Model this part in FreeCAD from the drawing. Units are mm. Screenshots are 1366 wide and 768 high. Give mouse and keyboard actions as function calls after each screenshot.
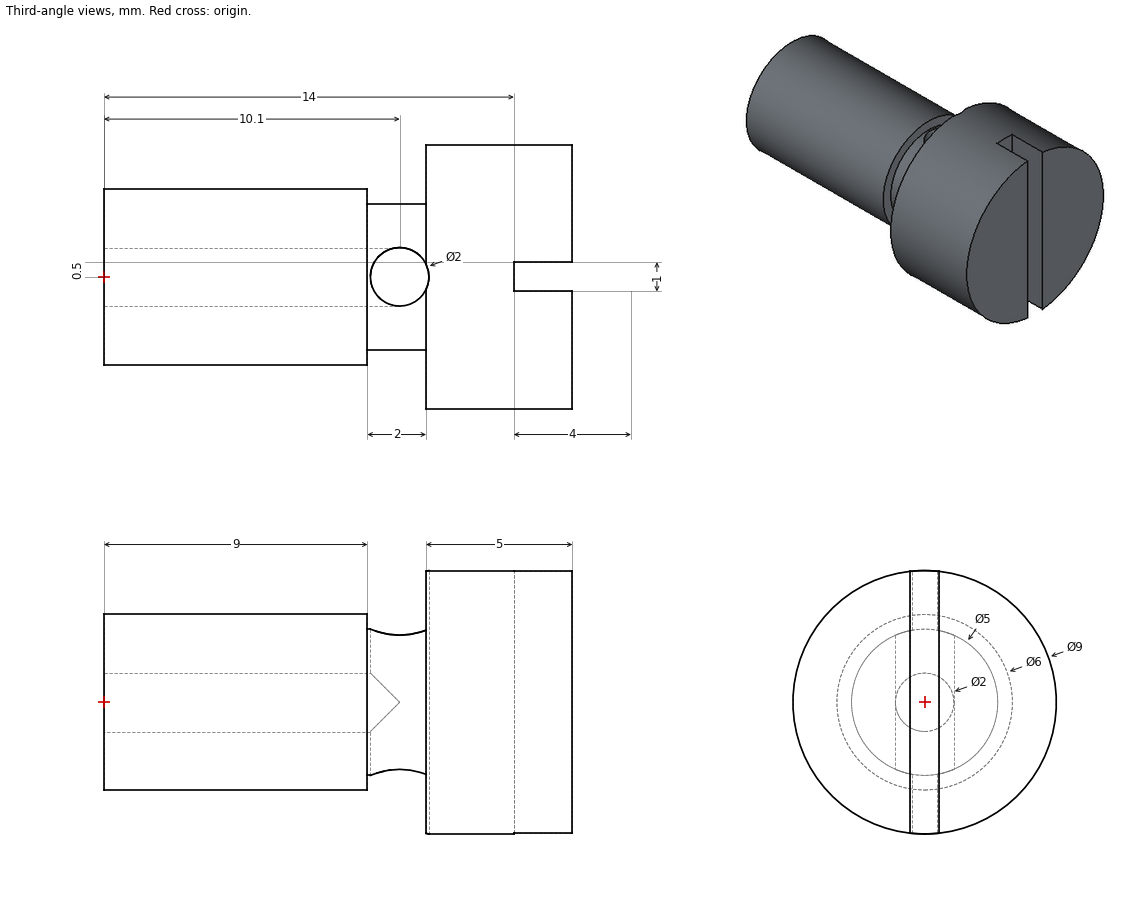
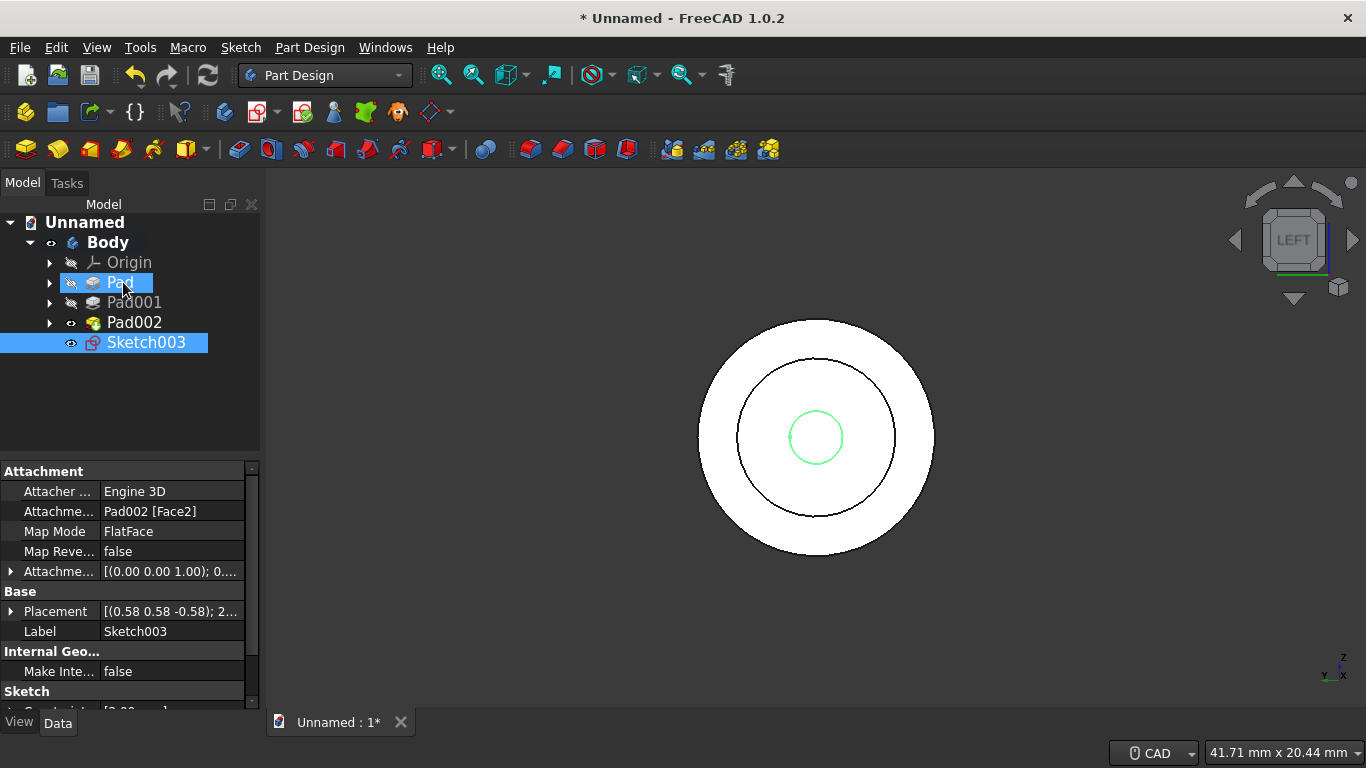
click(240, 150)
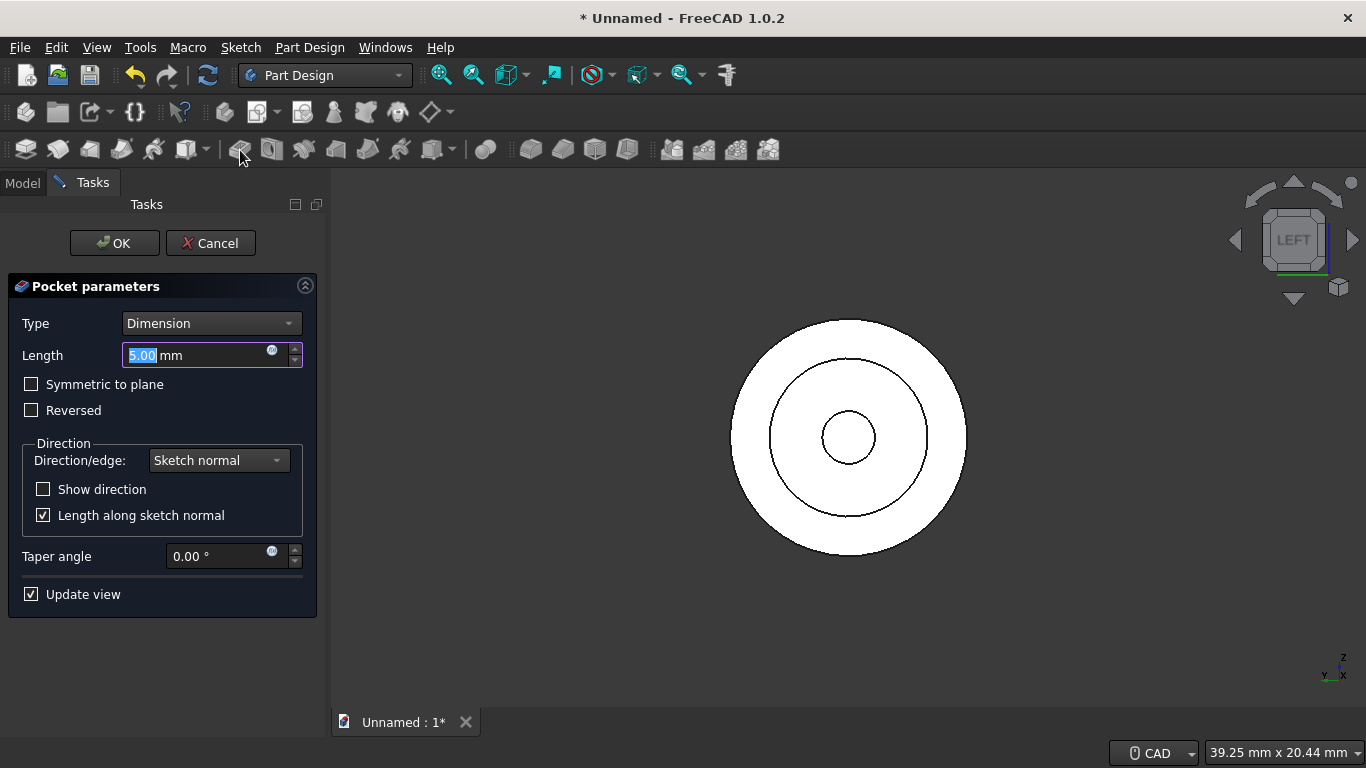
click(212, 324)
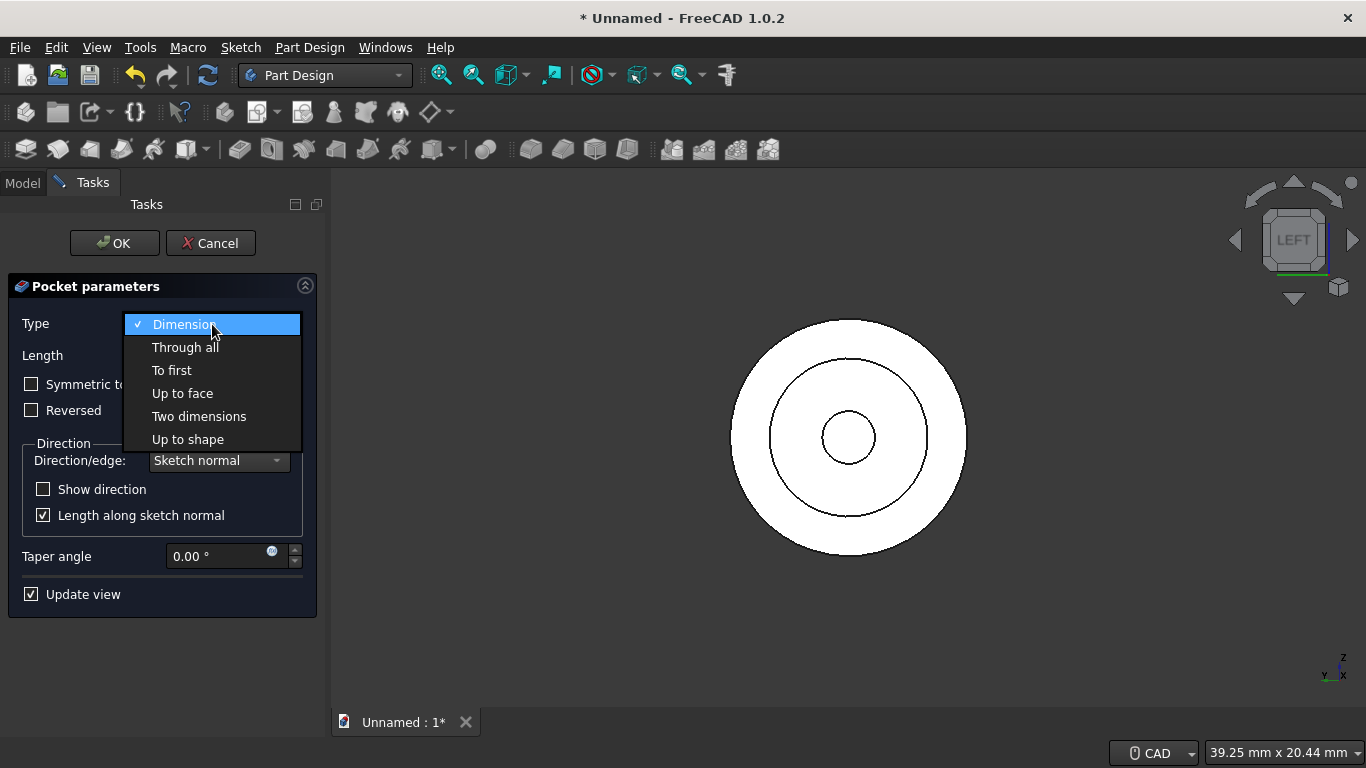
click(212, 416)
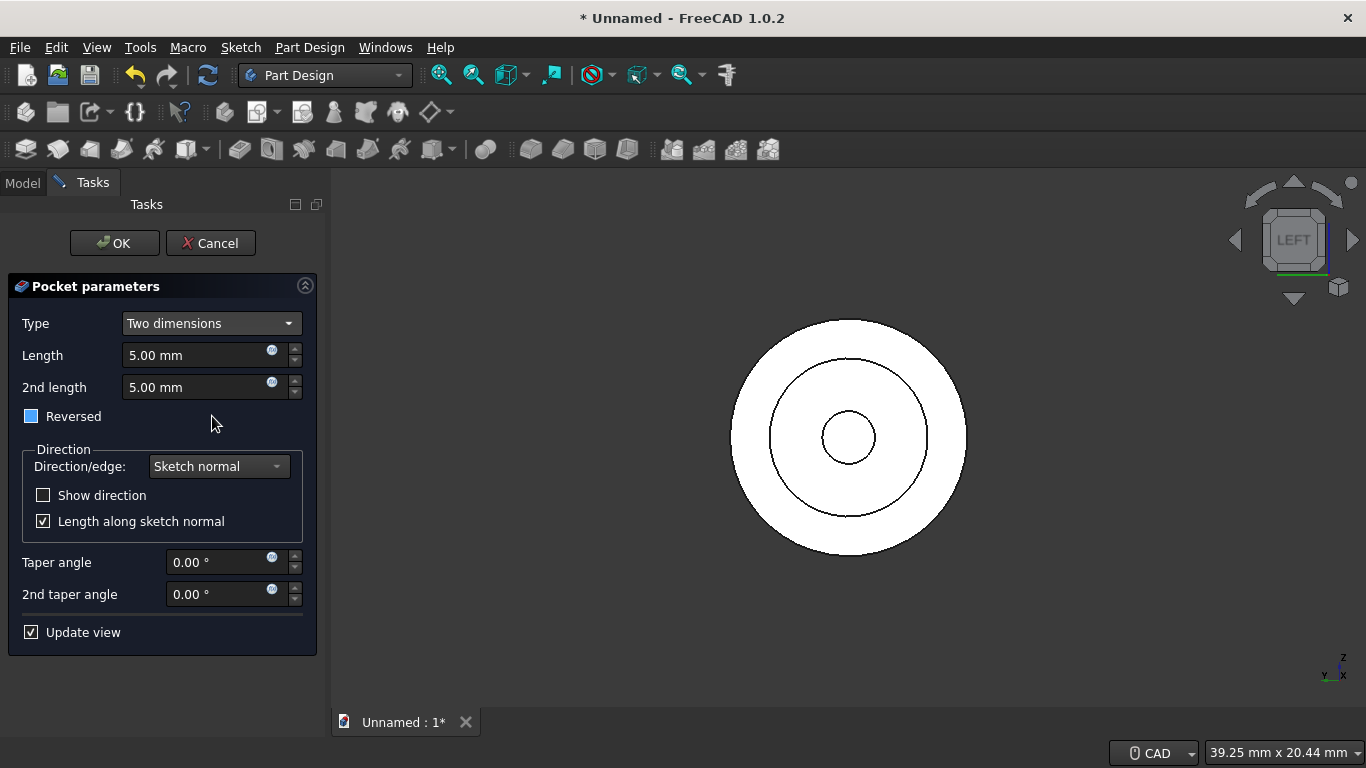
triple_click(204, 355)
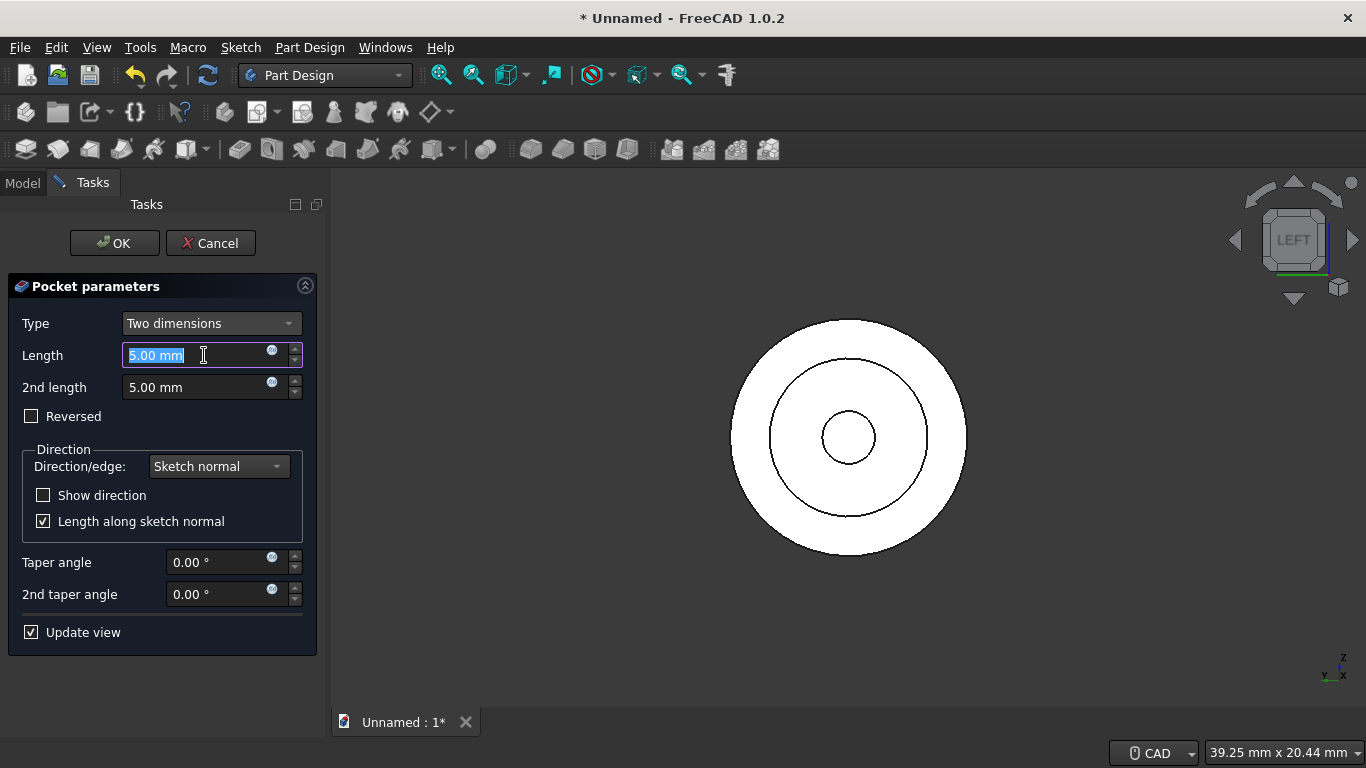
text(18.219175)
key(Tab)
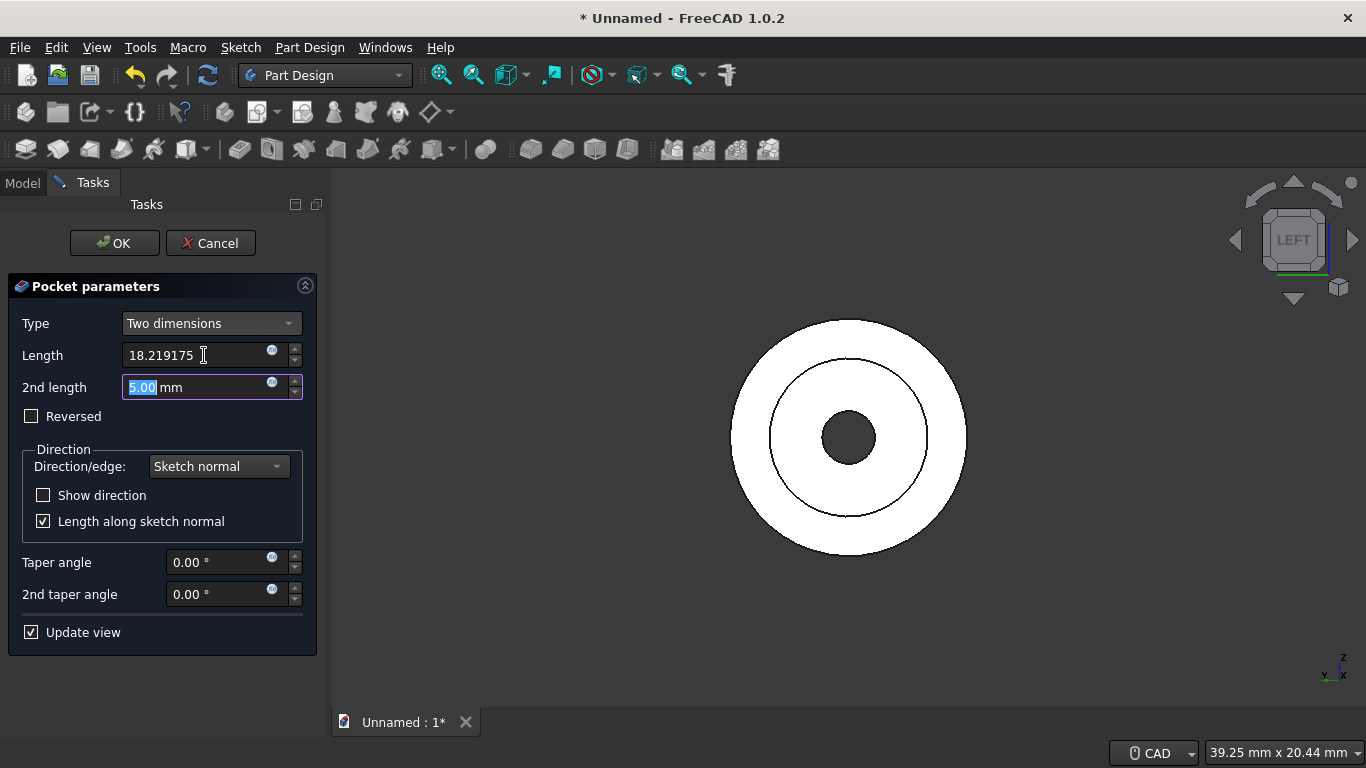
text(10.1)
key(Tab)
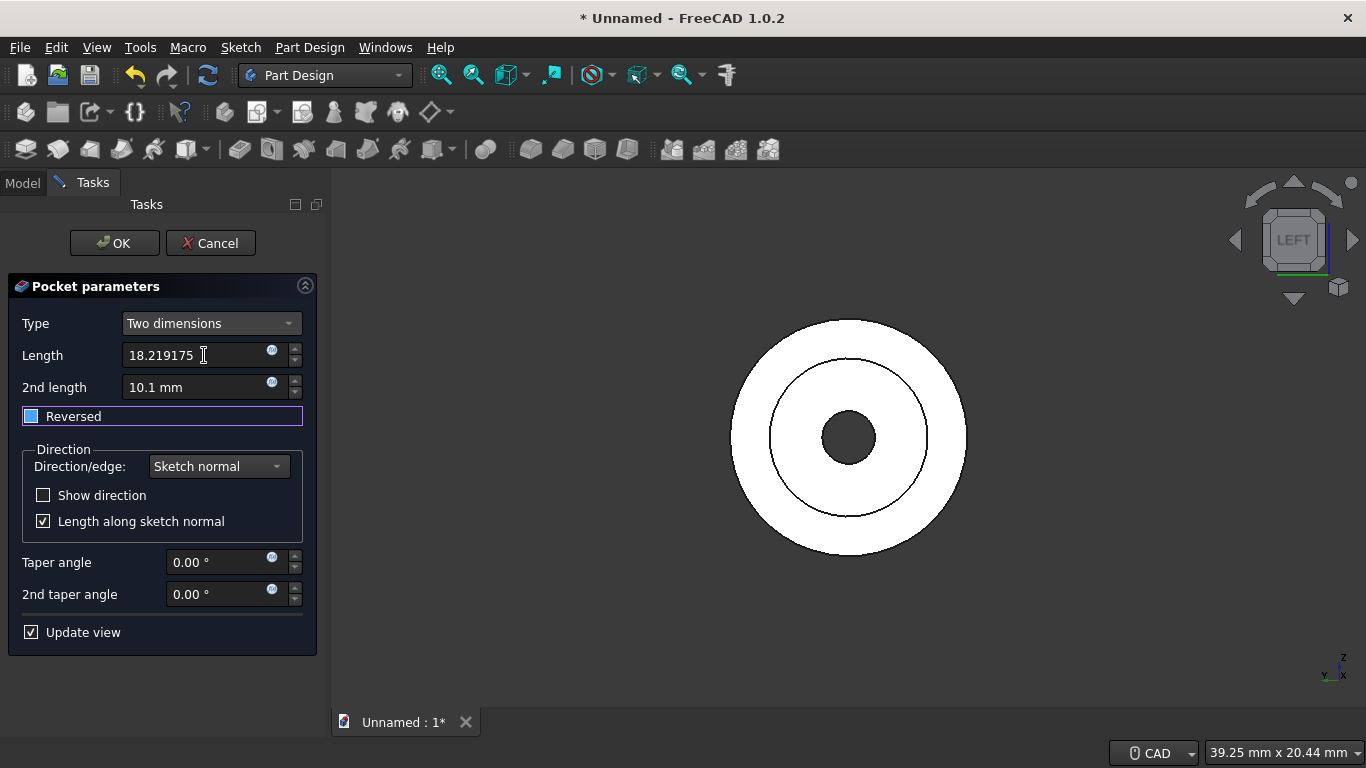
click(30, 416)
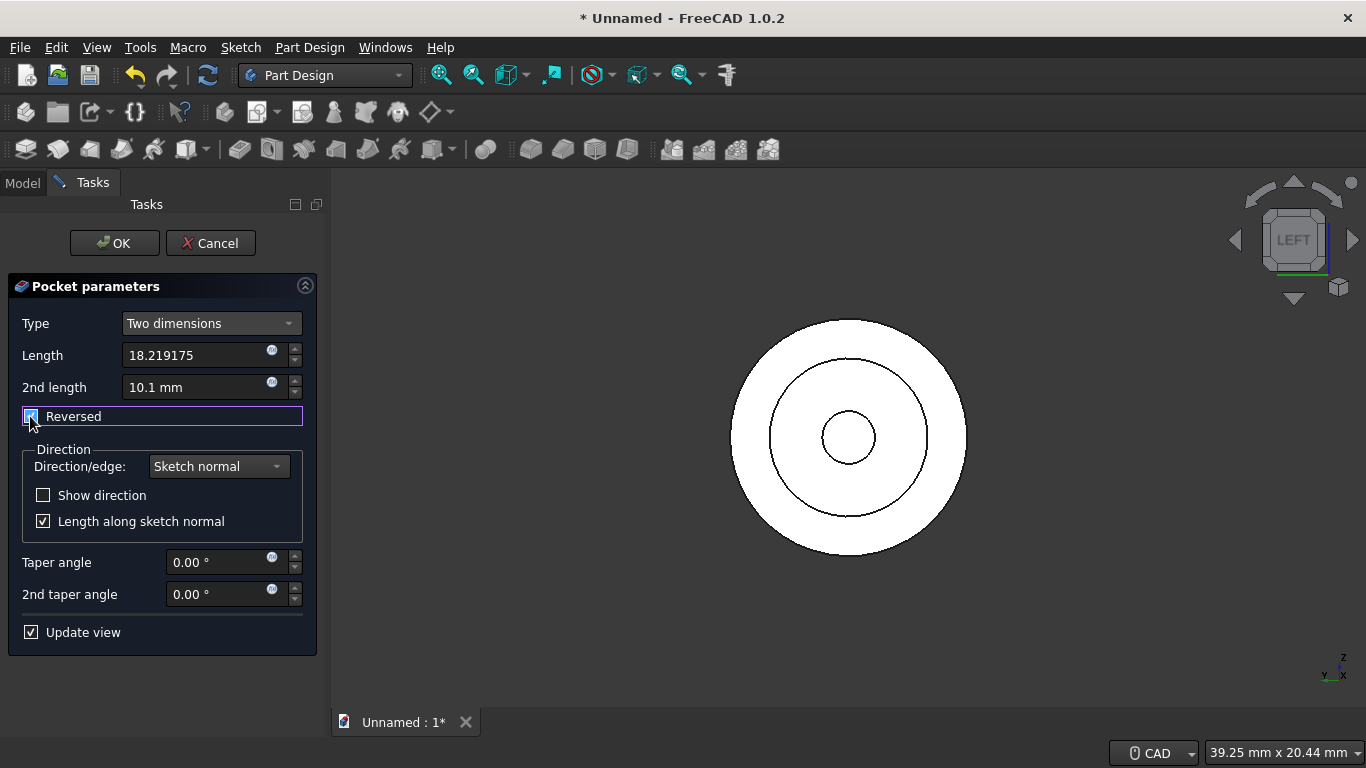
click(115, 243)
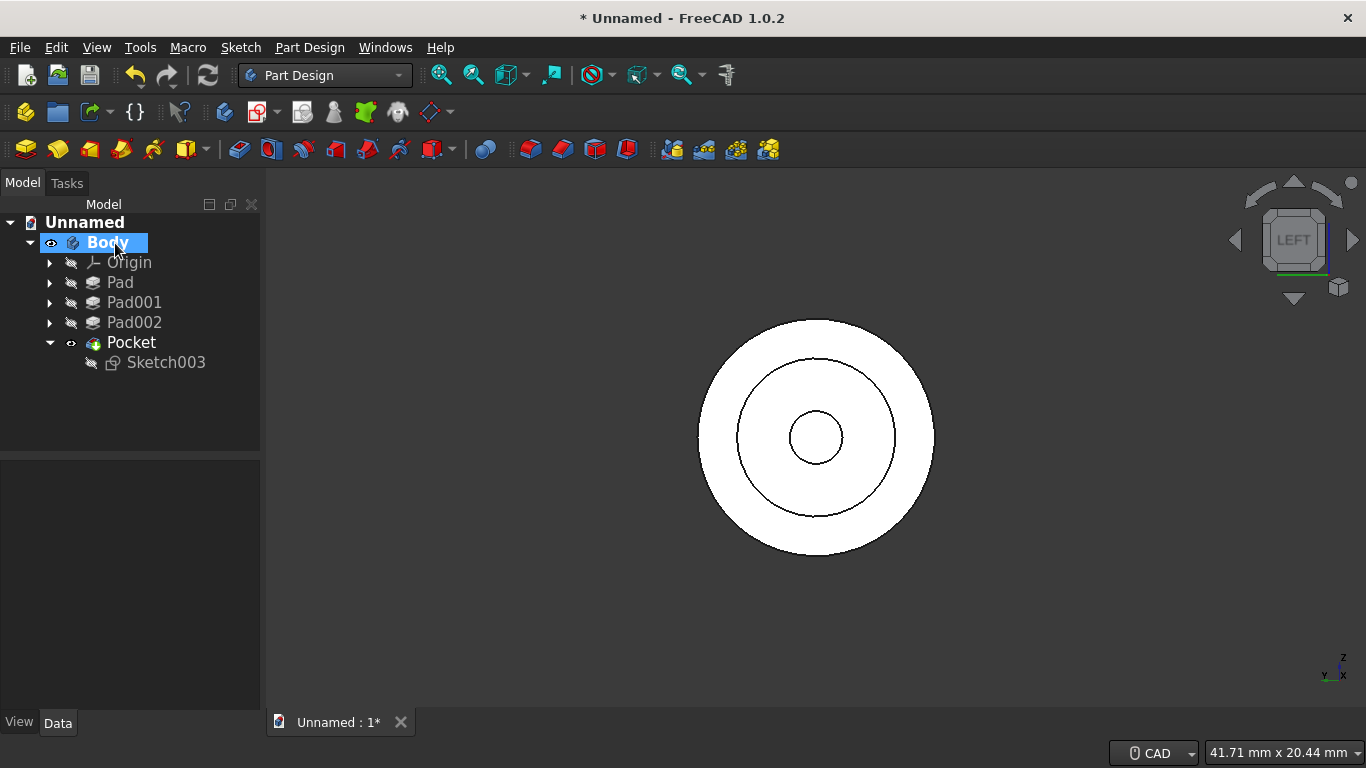
click(442, 76)